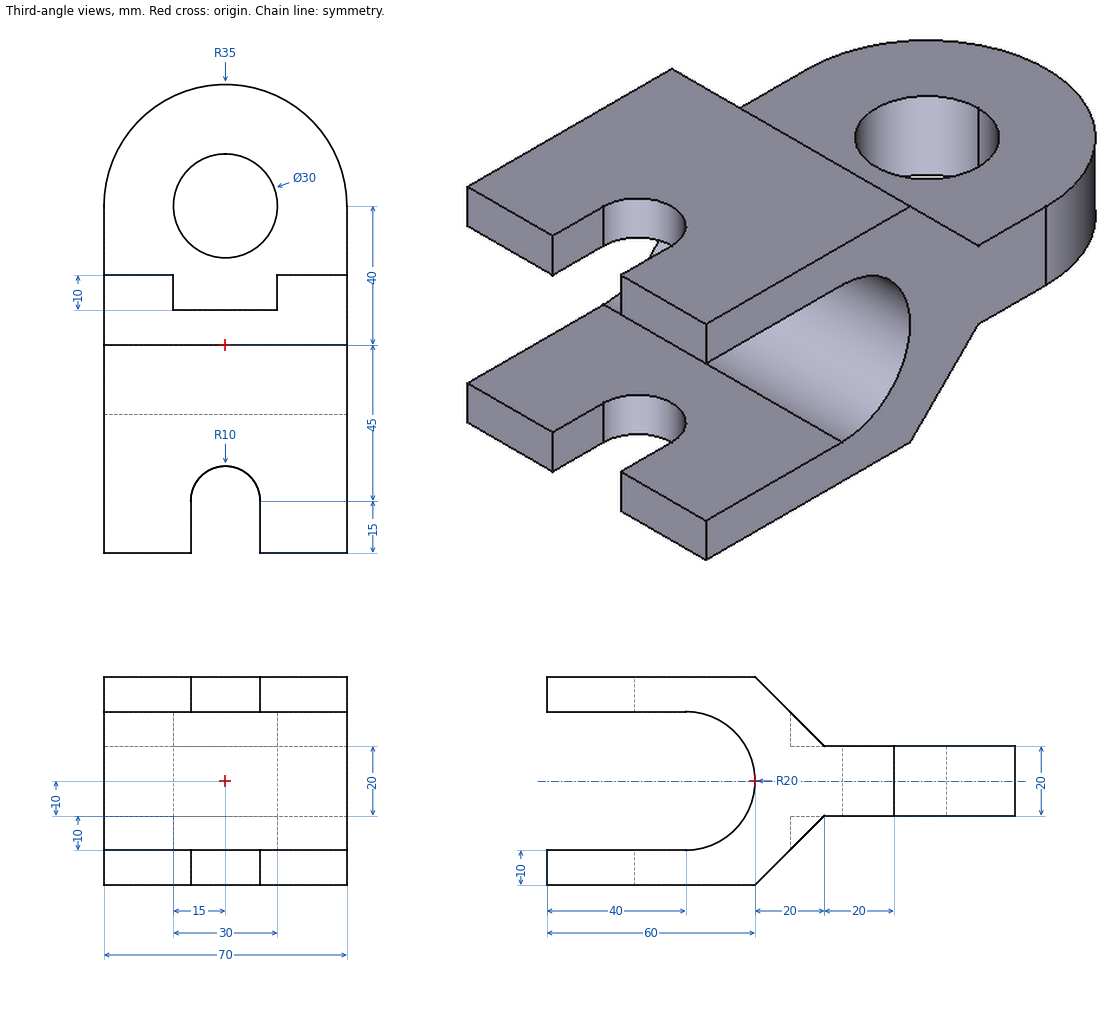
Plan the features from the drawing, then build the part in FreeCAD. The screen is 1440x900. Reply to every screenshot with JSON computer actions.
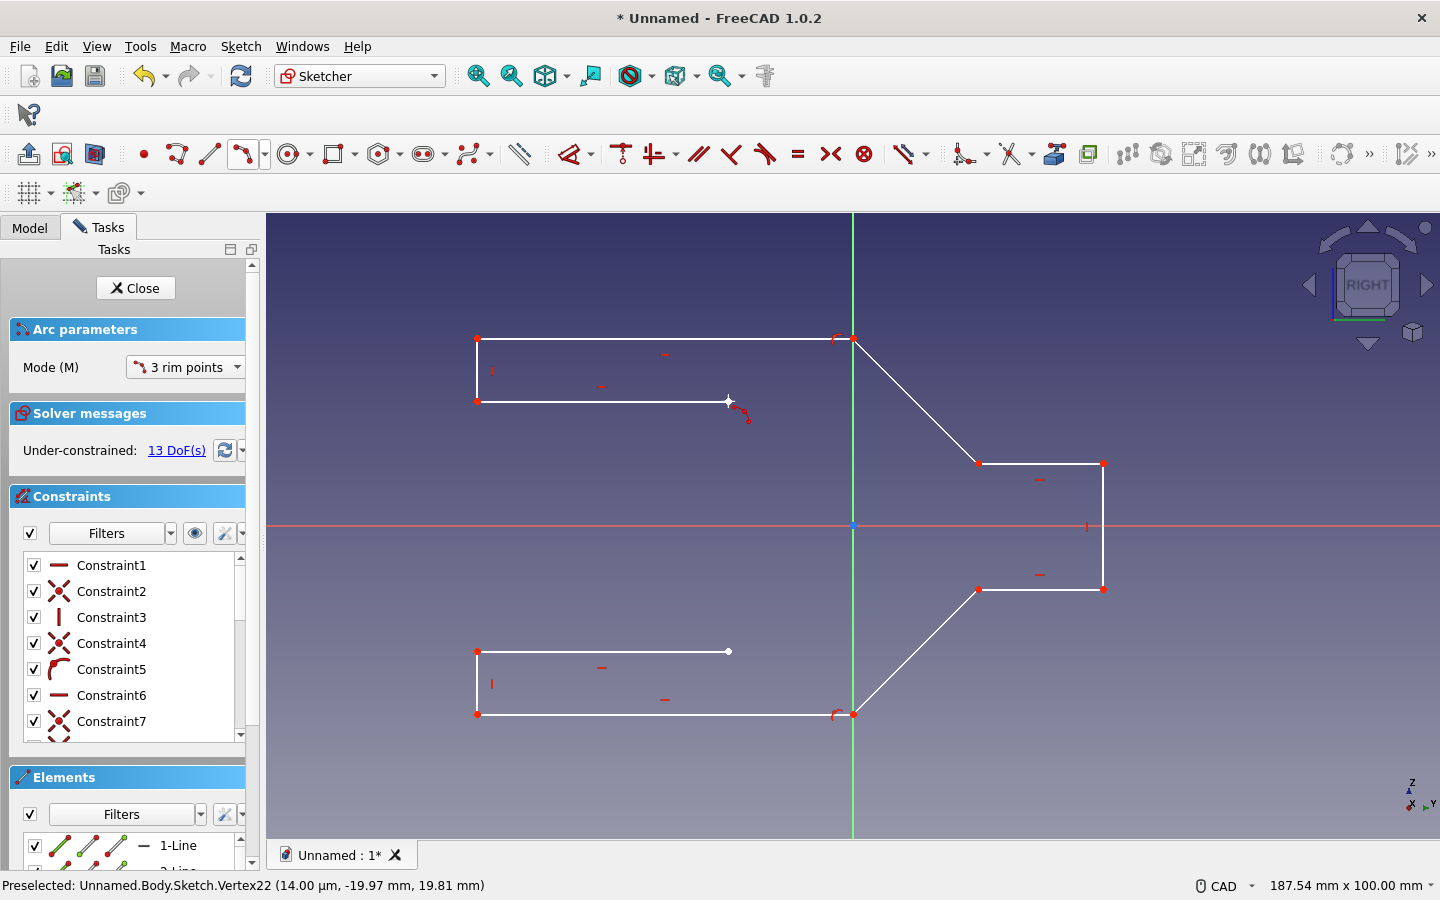
{"action": "left_click", "coordinate": [728, 402]}
{"action": "left_click", "coordinate": [728, 652]}
{"action": "left_click", "coordinate": [829, 600]}
{"action": "key", "text": "Escape"}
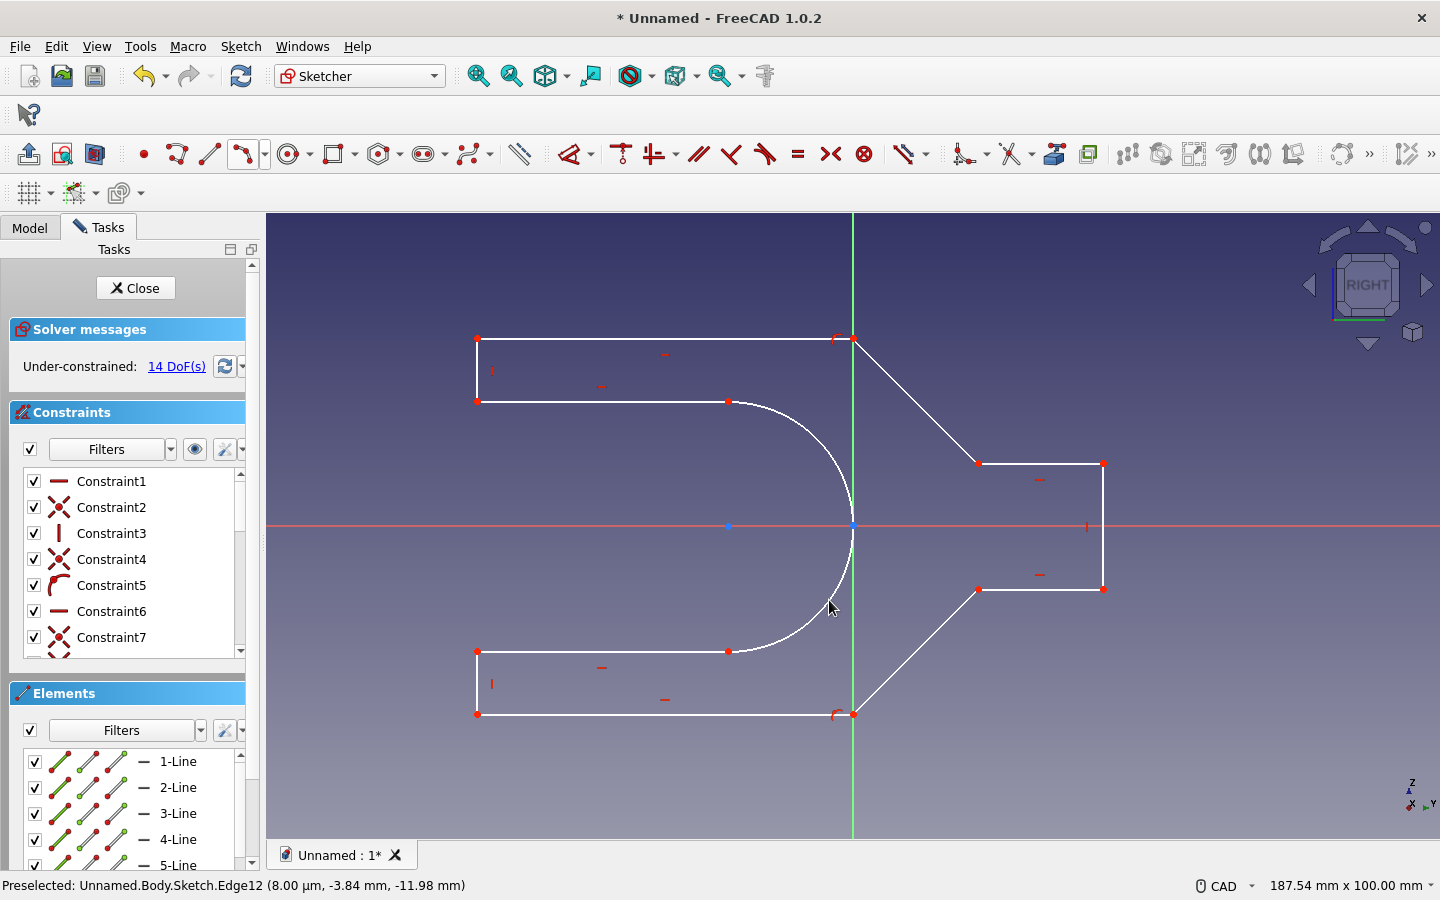
{"action": "left_click", "coordinate": [653, 652]}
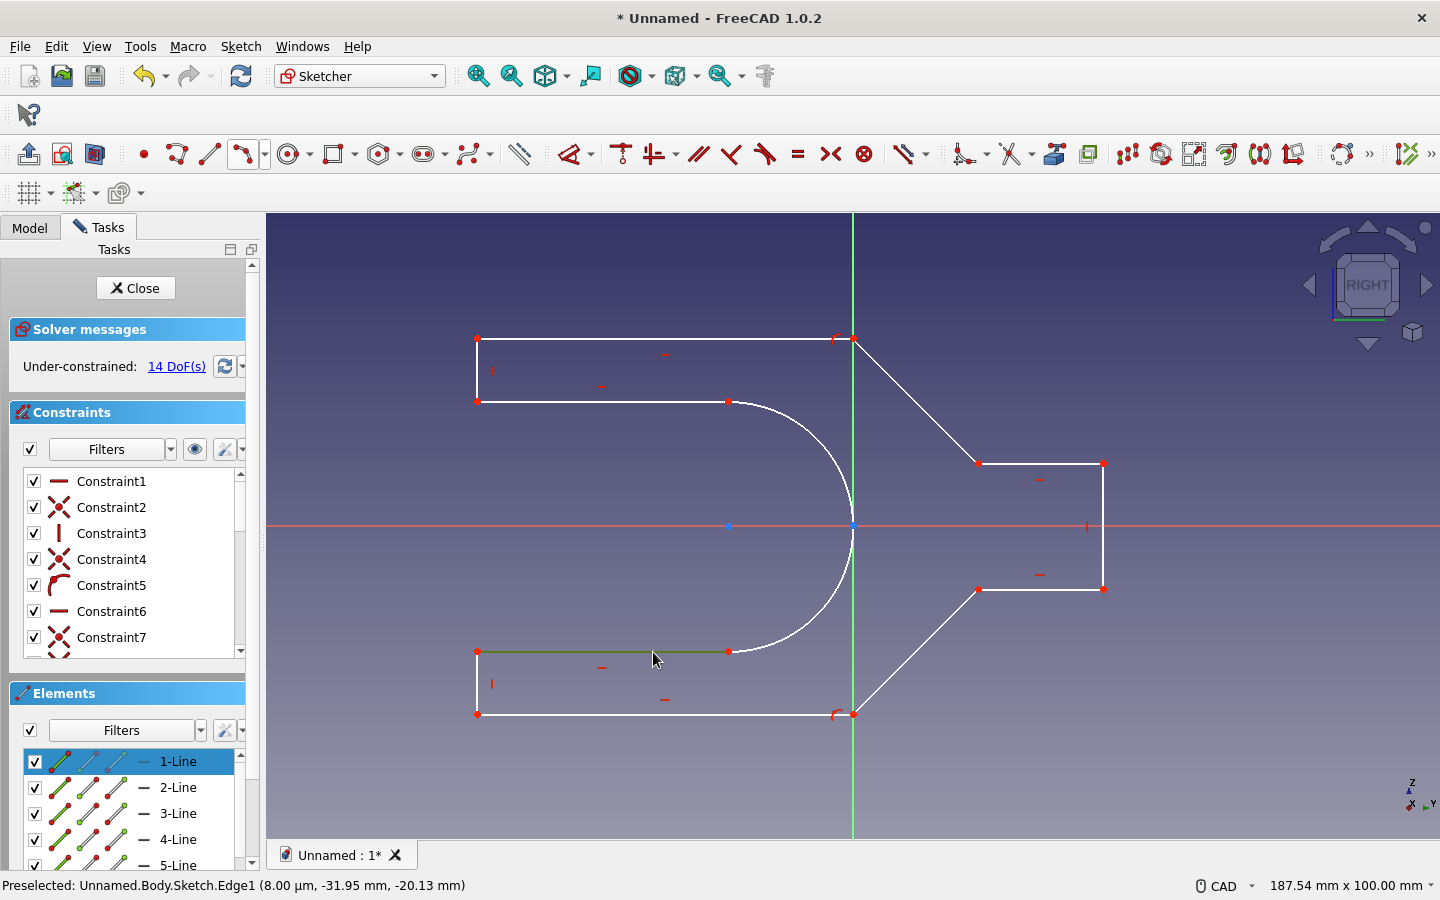
{"action": "left_click", "coordinate": [829, 601]}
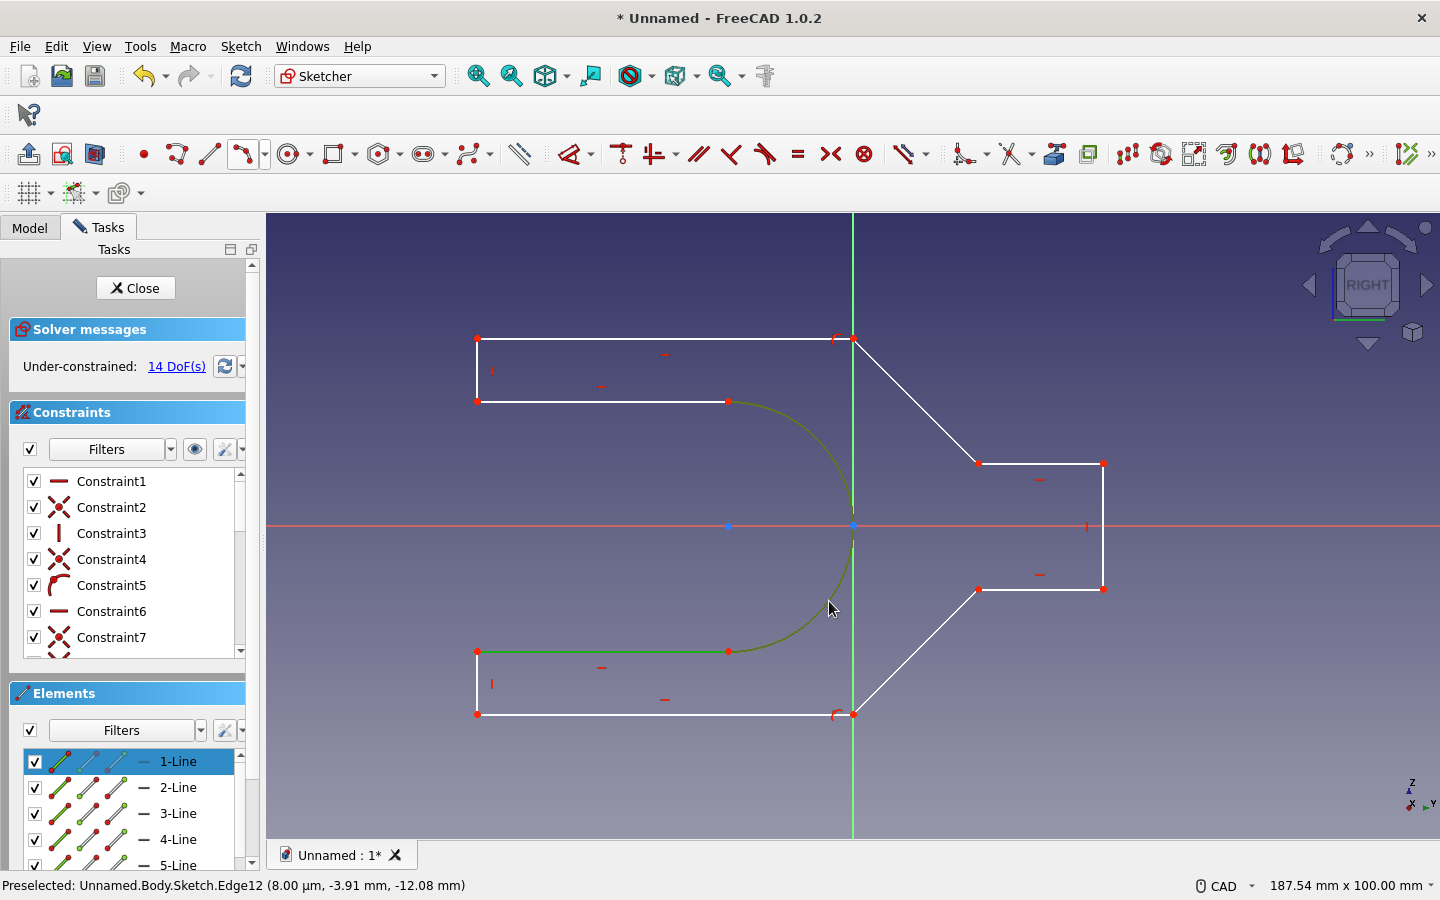
{"action": "key", "text": "t"}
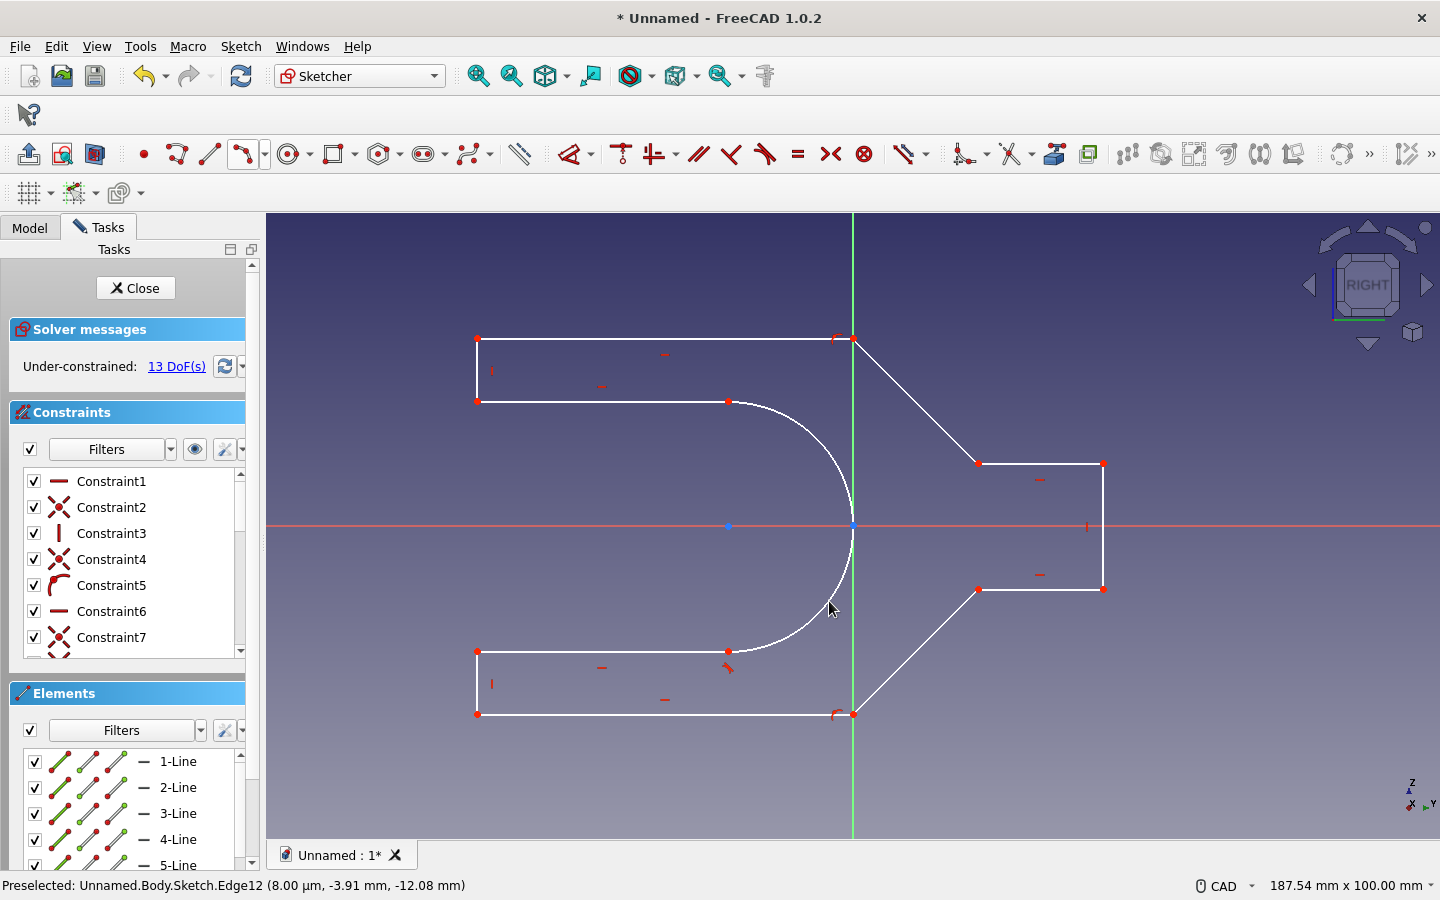
{"action": "left_click", "coordinate": [552, 402]}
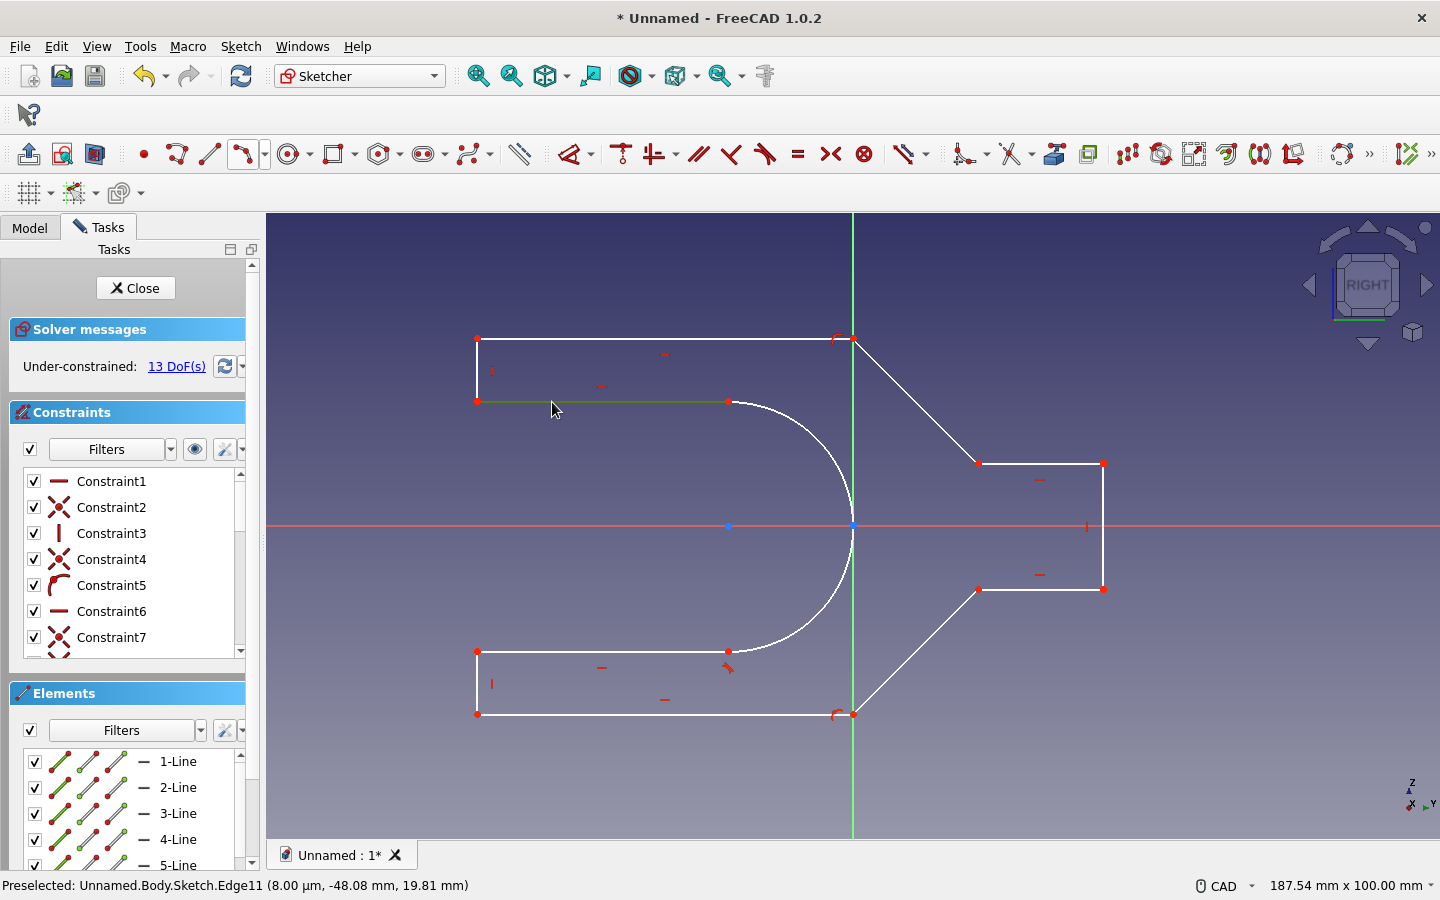
{"action": "left_click", "coordinate": [829, 600]}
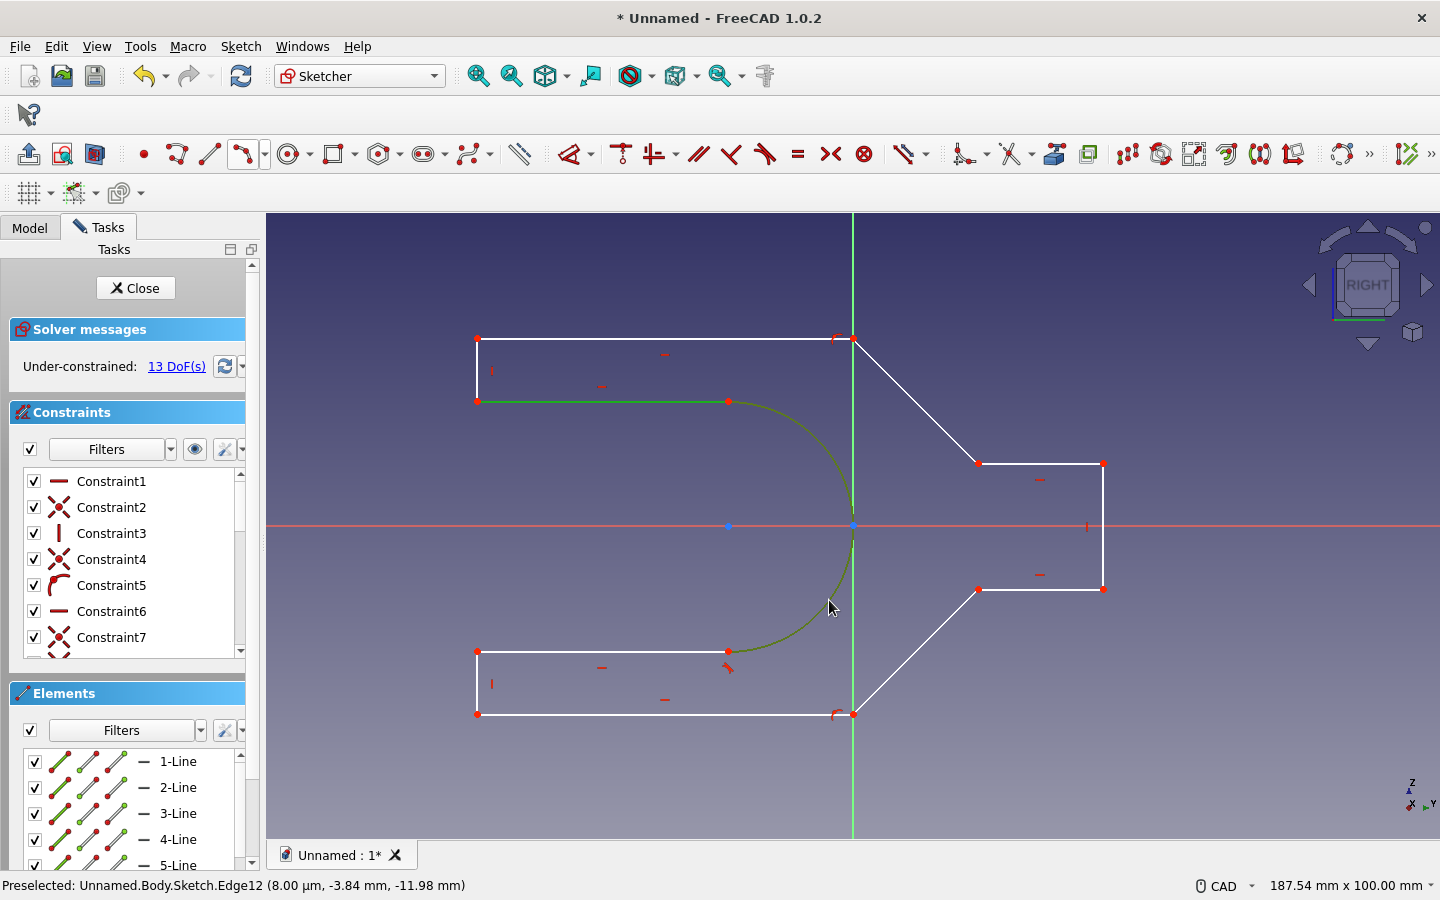
{"action": "key", "text": "t"}